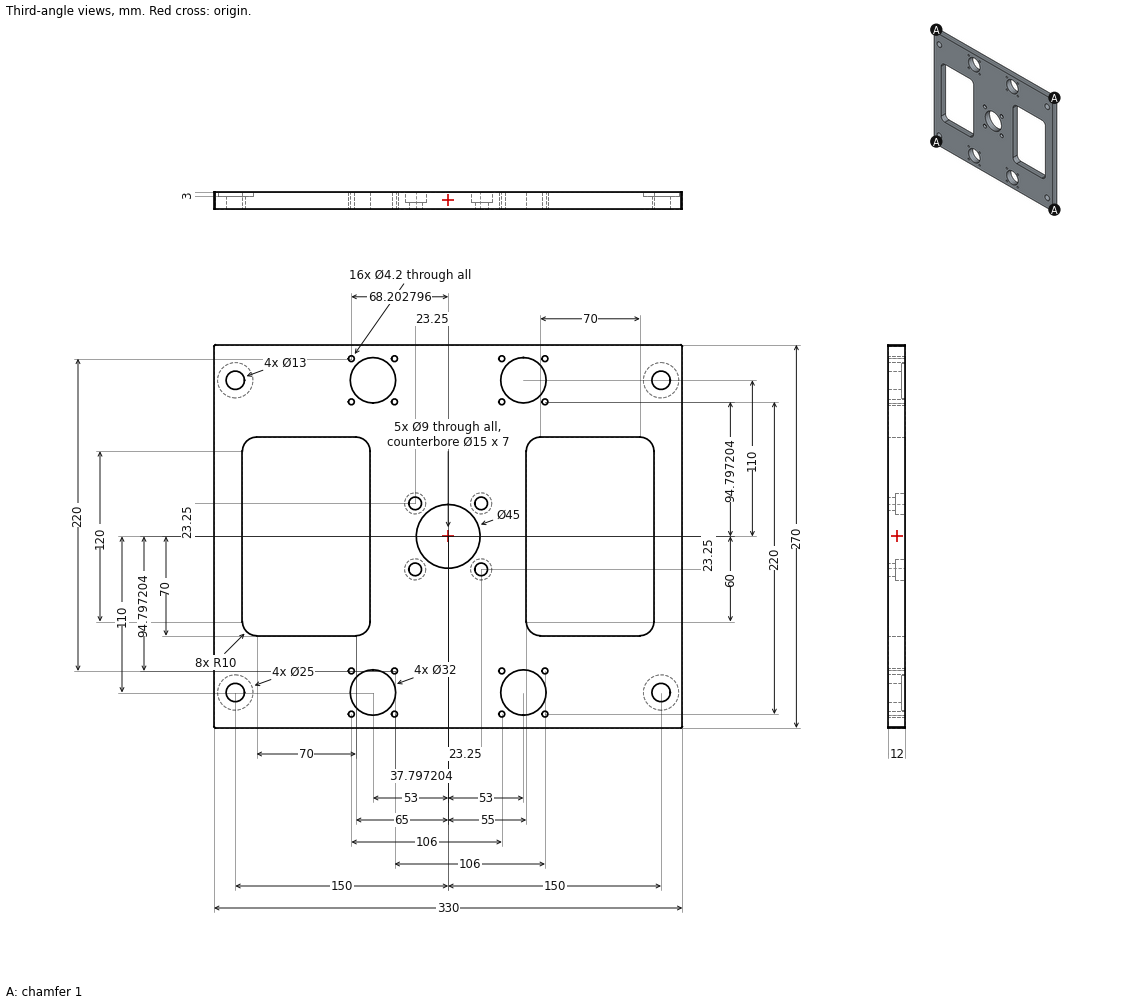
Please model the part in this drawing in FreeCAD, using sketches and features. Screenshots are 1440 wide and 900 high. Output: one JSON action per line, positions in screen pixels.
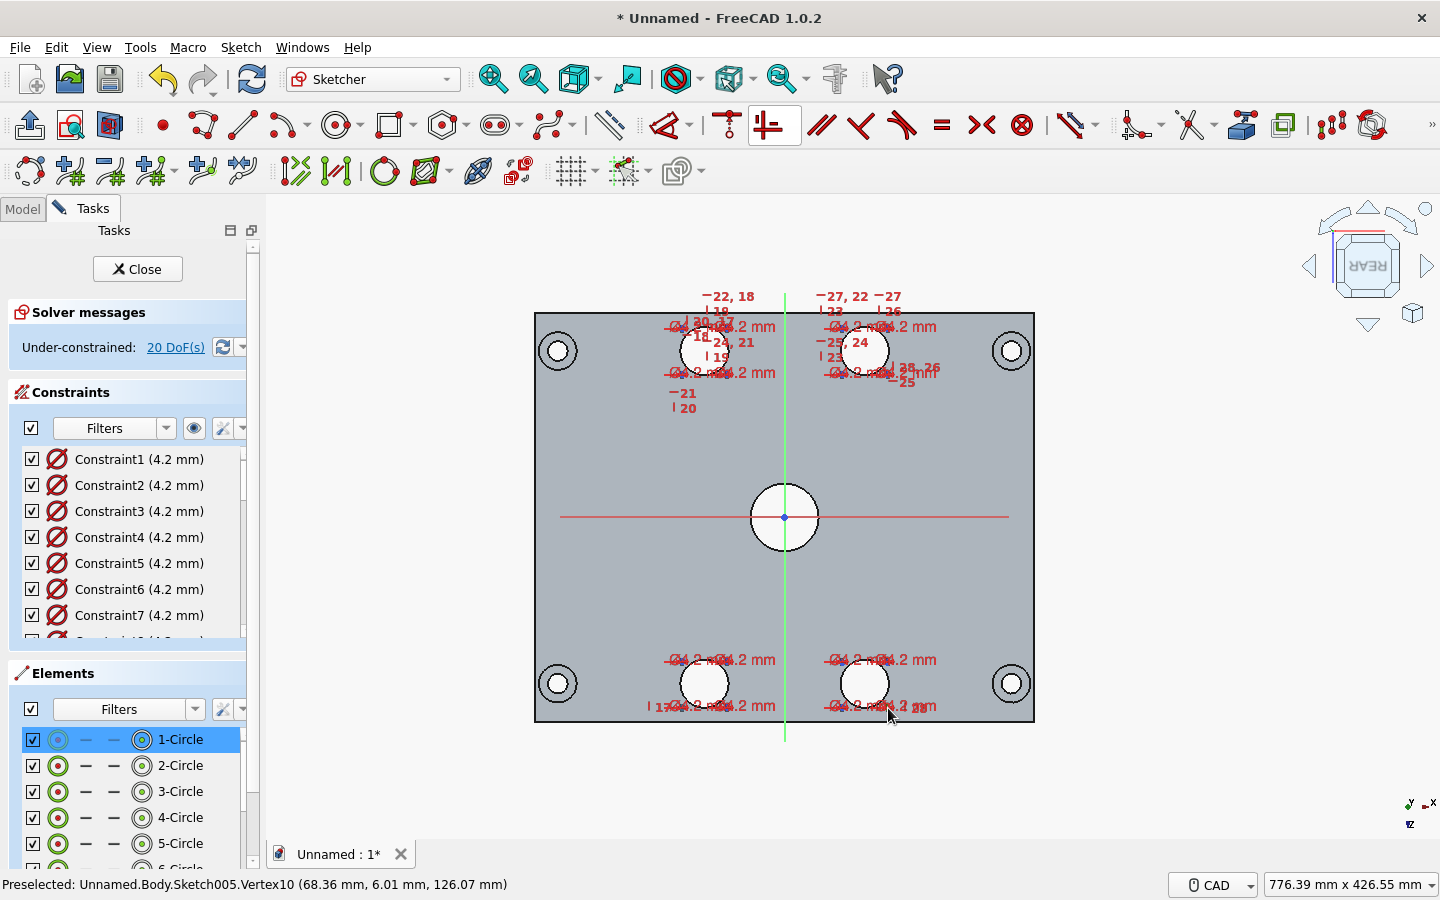
{"action": "left_click", "coordinate": [796, 126]}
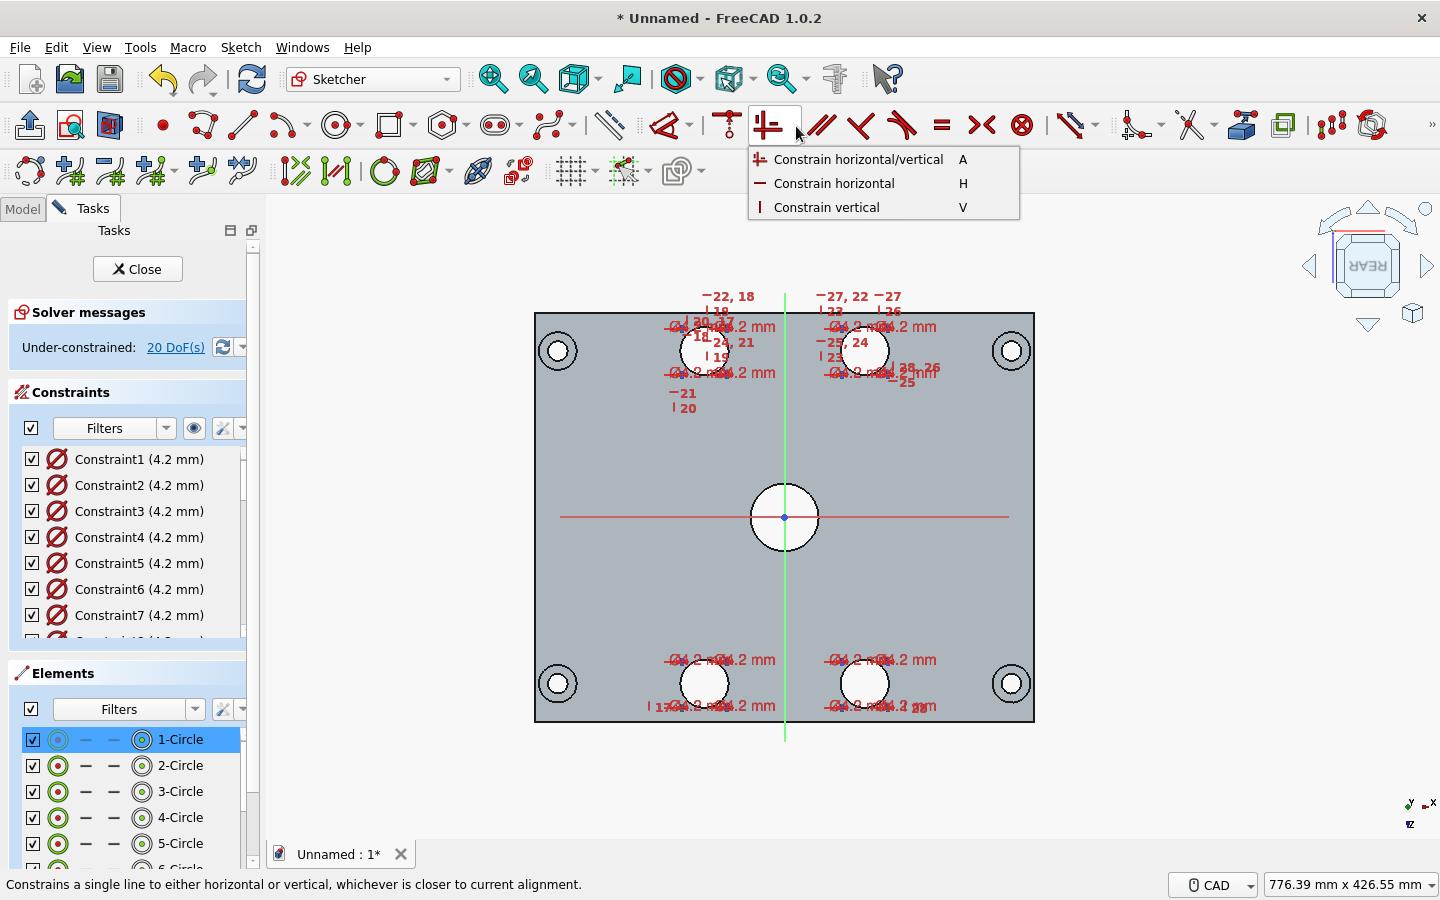
{"action": "left_click", "coordinate": [884, 183]}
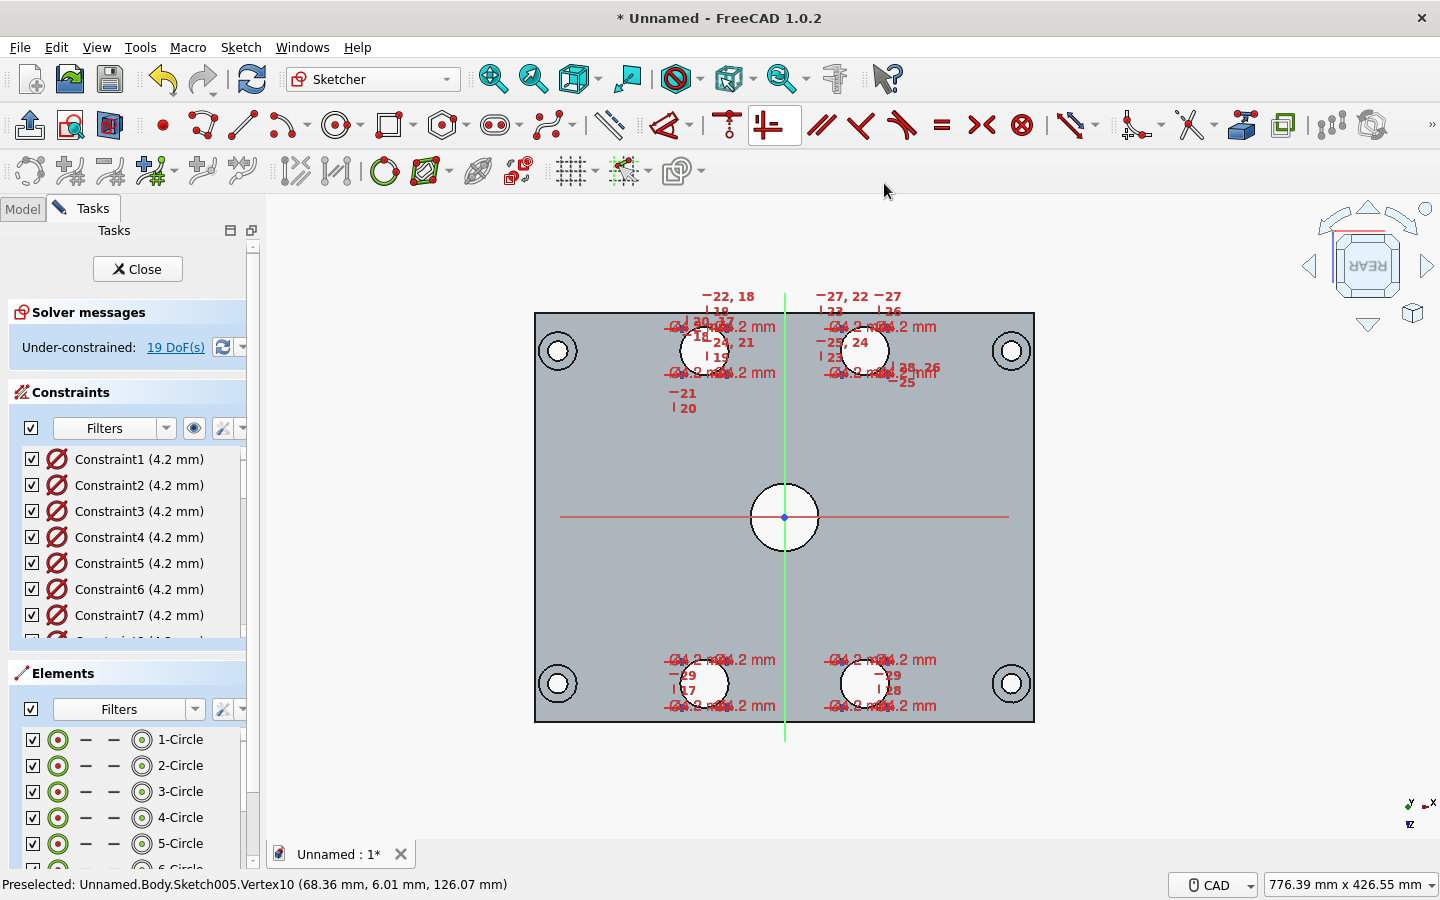
{"action": "left_click", "coordinate": [888, 708]}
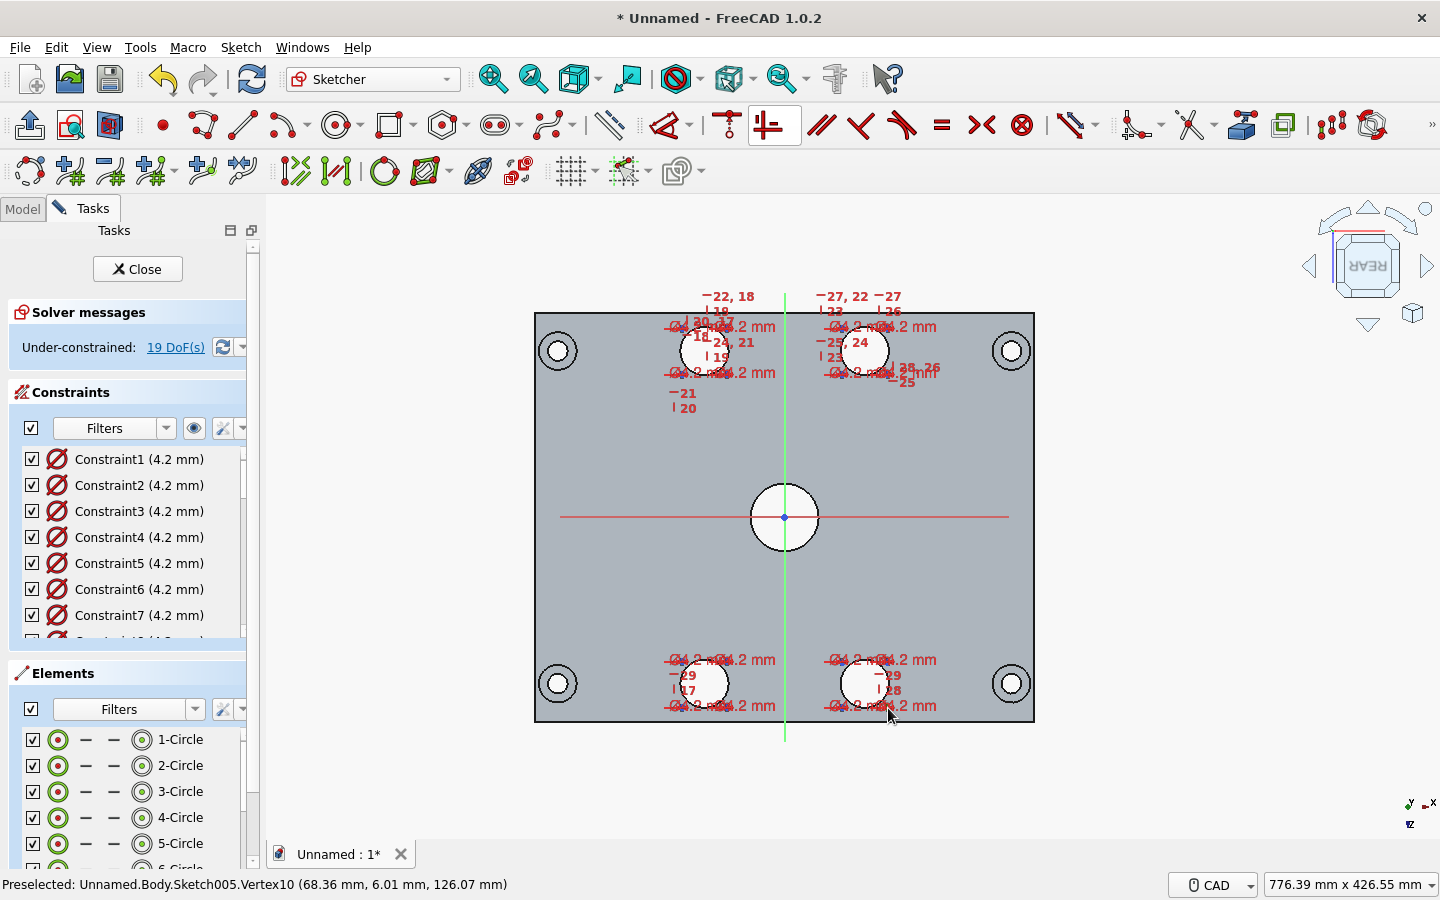
{"action": "left_click", "coordinate": [888, 662]}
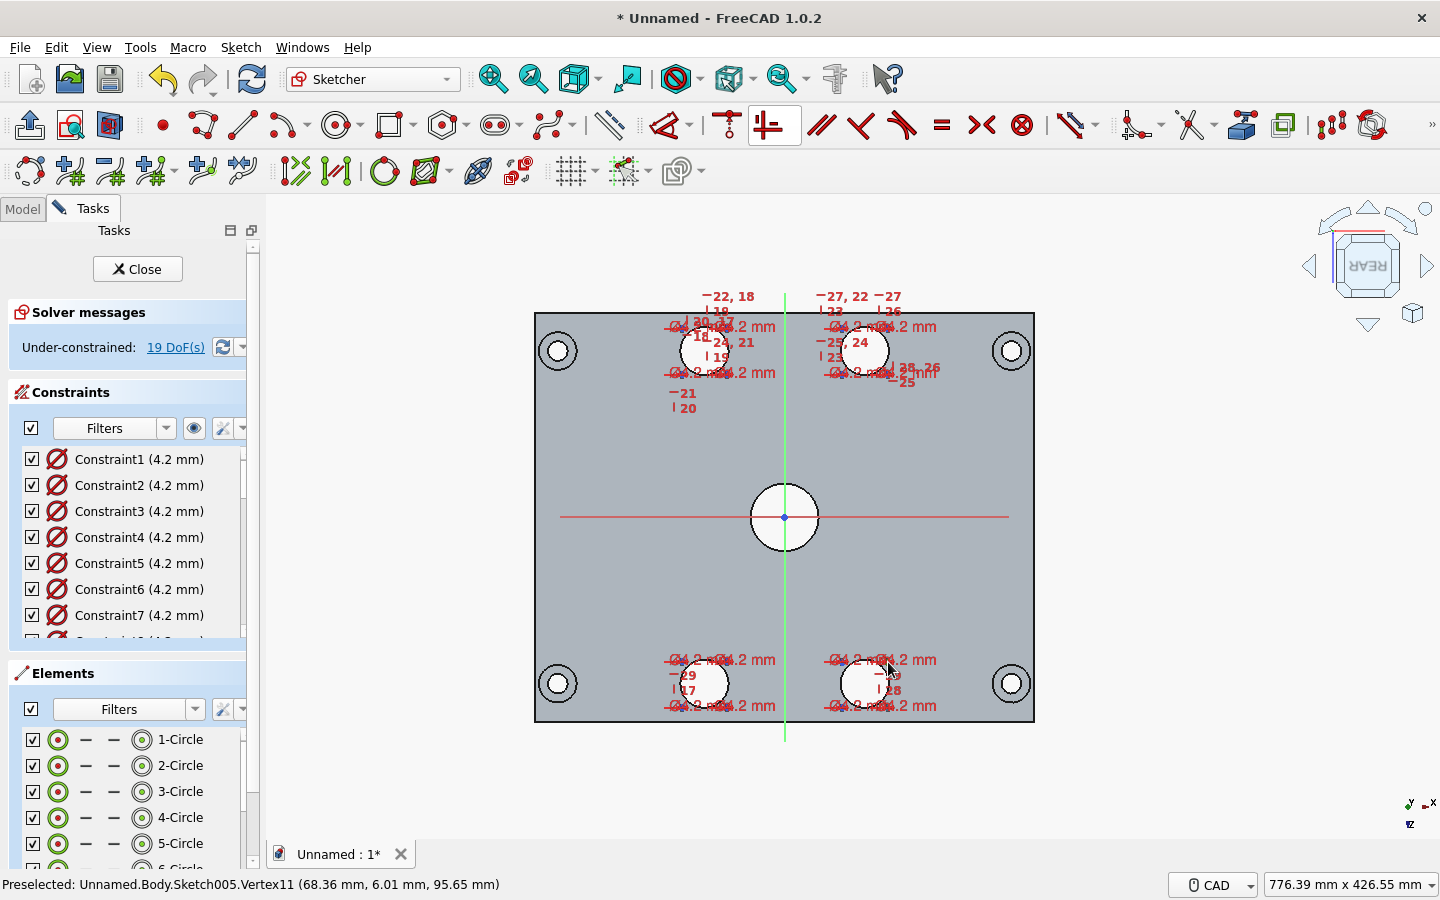
{"action": "left_click", "coordinate": [796, 126]}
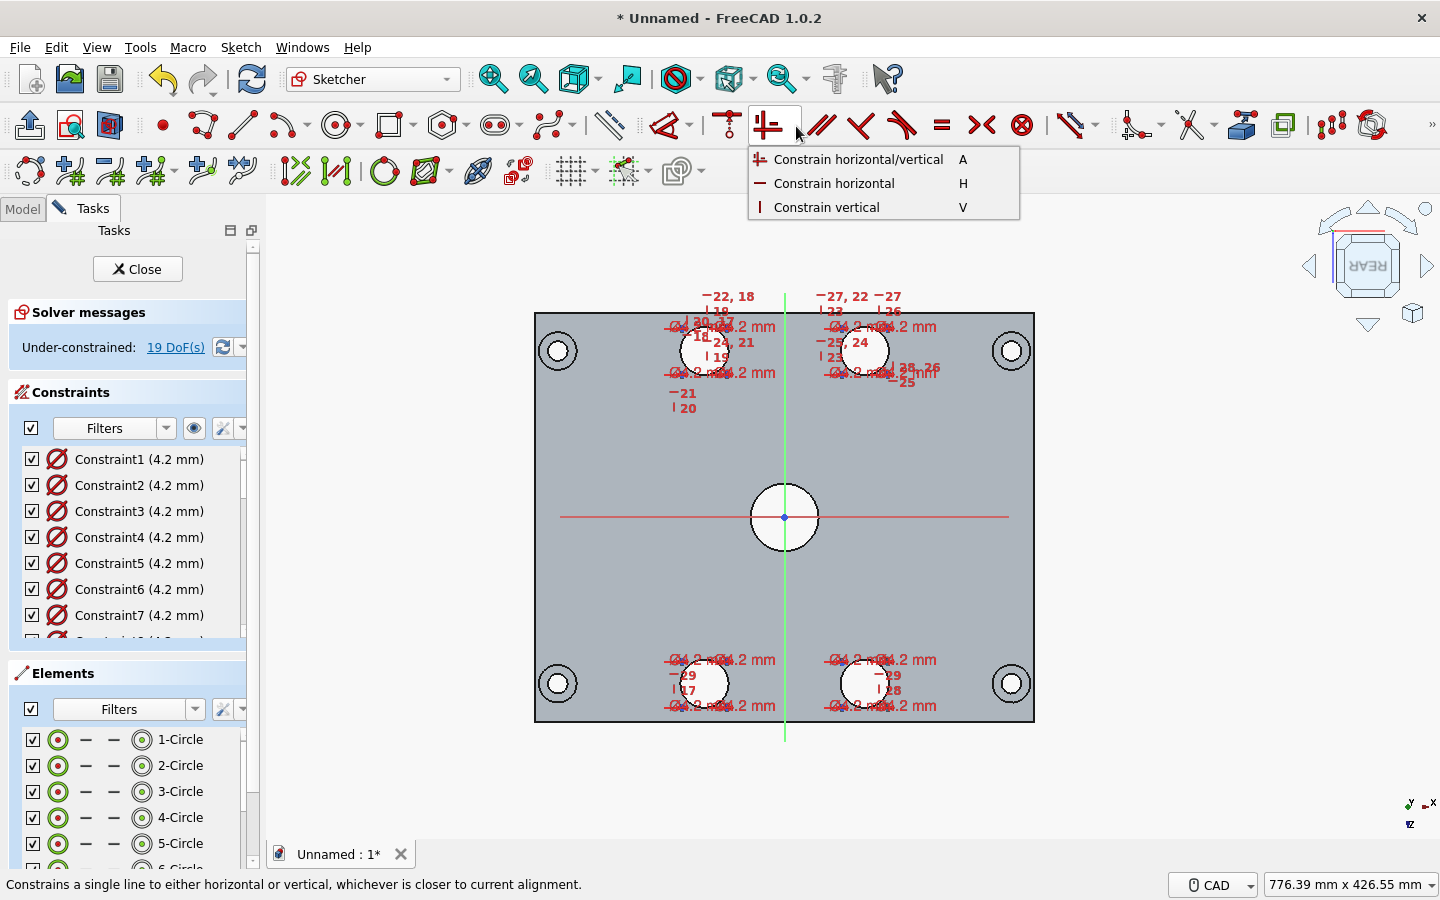
{"action": "left_click", "coordinate": [884, 207]}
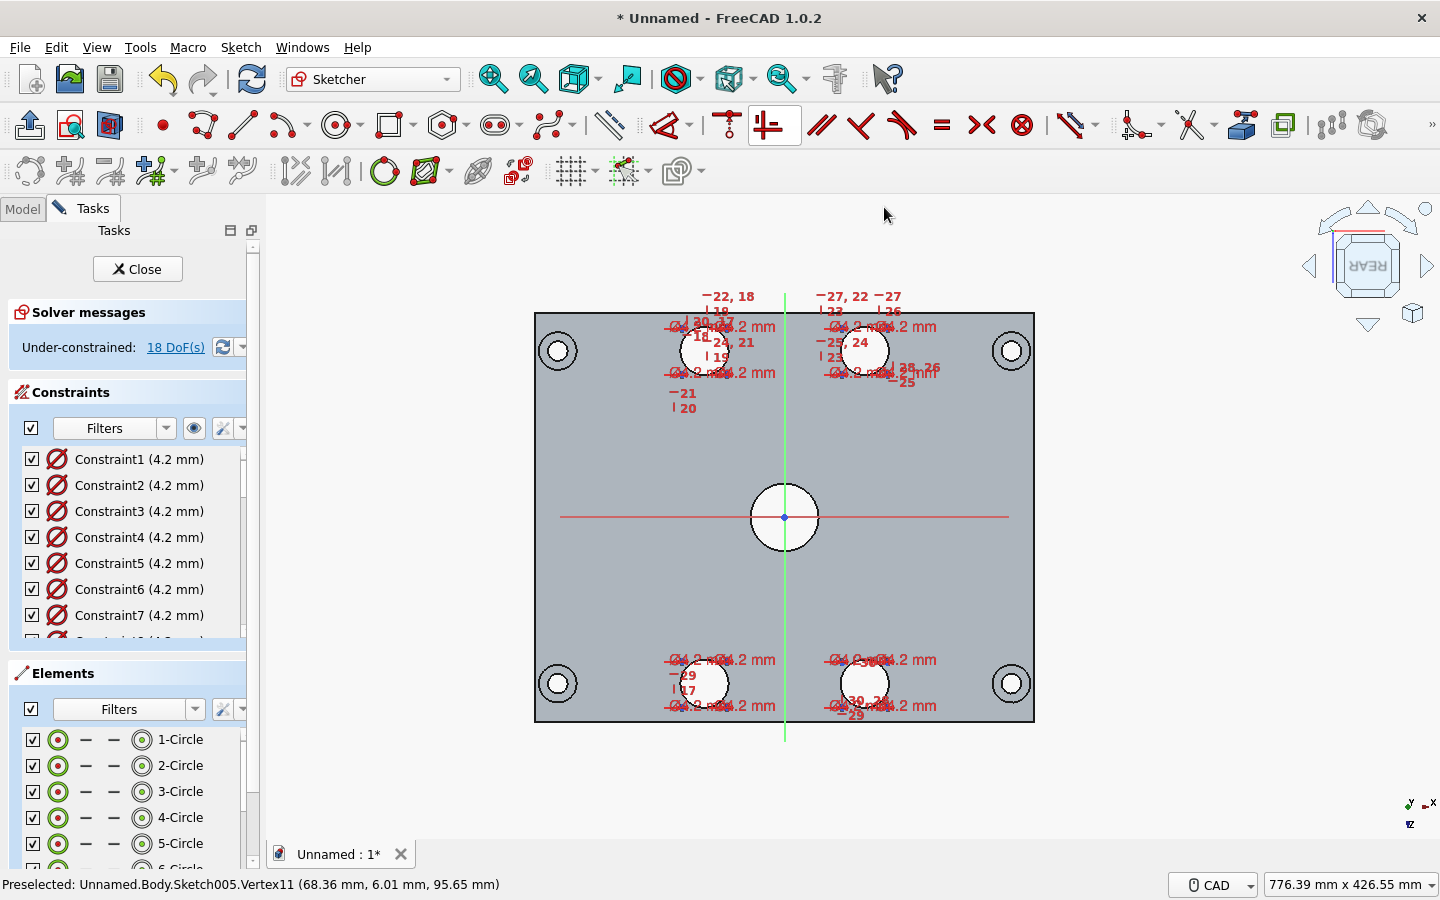
{"action": "left_click", "coordinate": [842, 375]}